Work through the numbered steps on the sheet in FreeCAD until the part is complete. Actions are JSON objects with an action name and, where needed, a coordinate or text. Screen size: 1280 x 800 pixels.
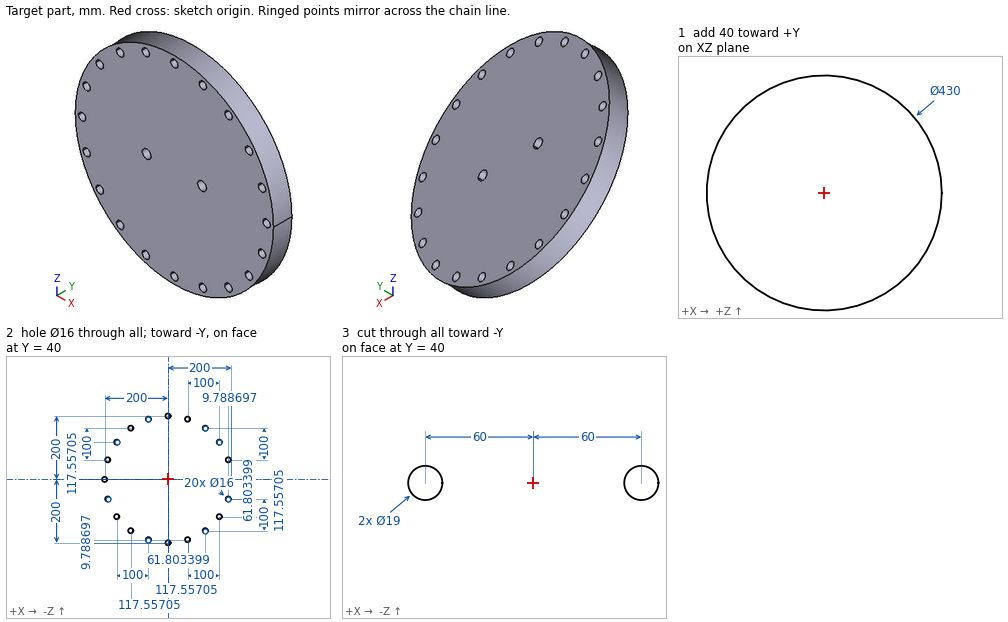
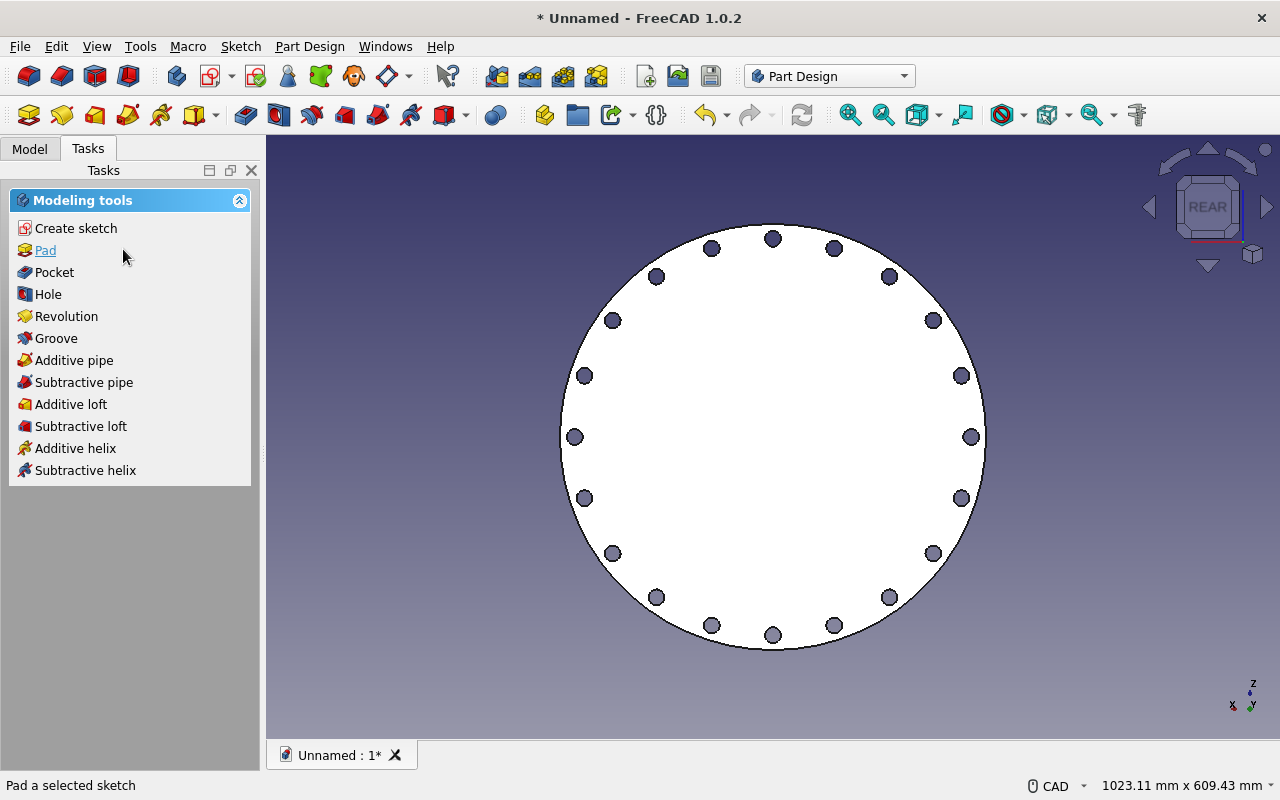
{"action": "left_click", "coordinate": [246, 116]}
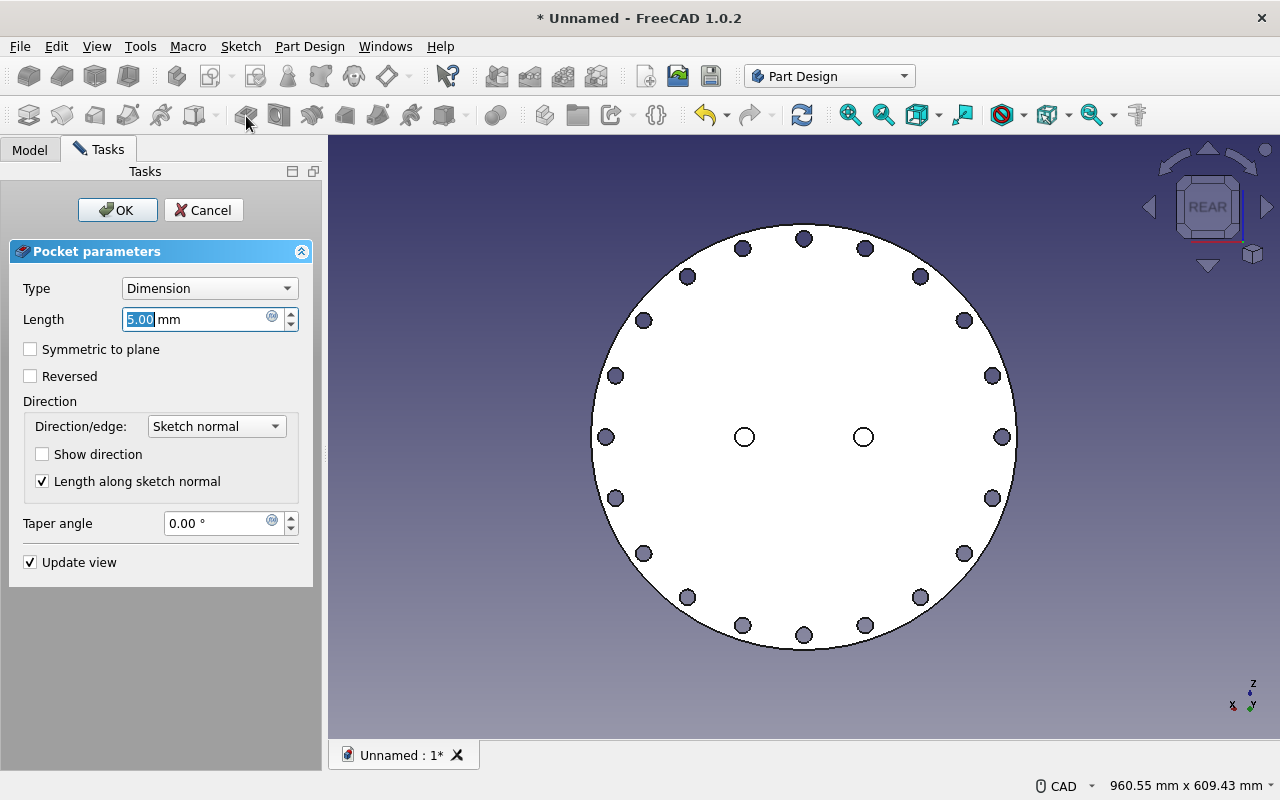
{"action": "left_click", "coordinate": [210, 288]}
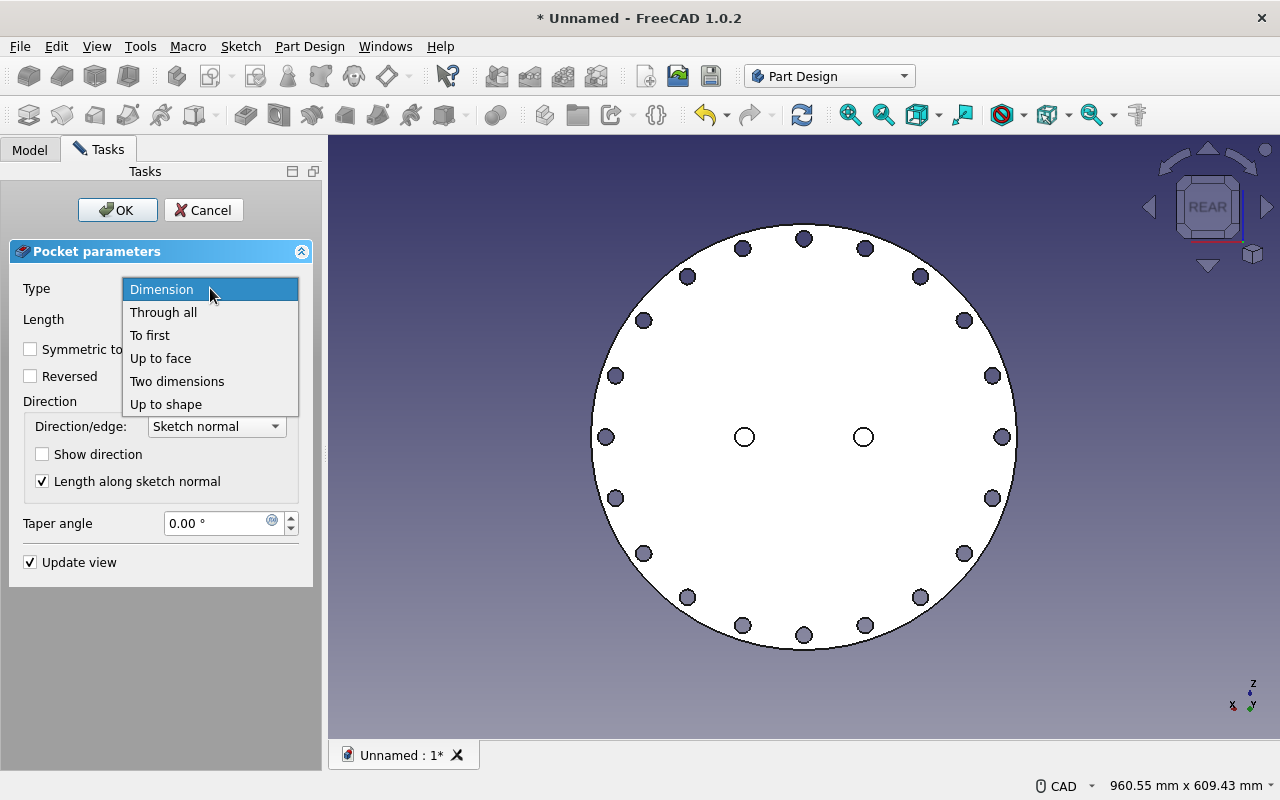
{"action": "left_click", "coordinate": [208, 312]}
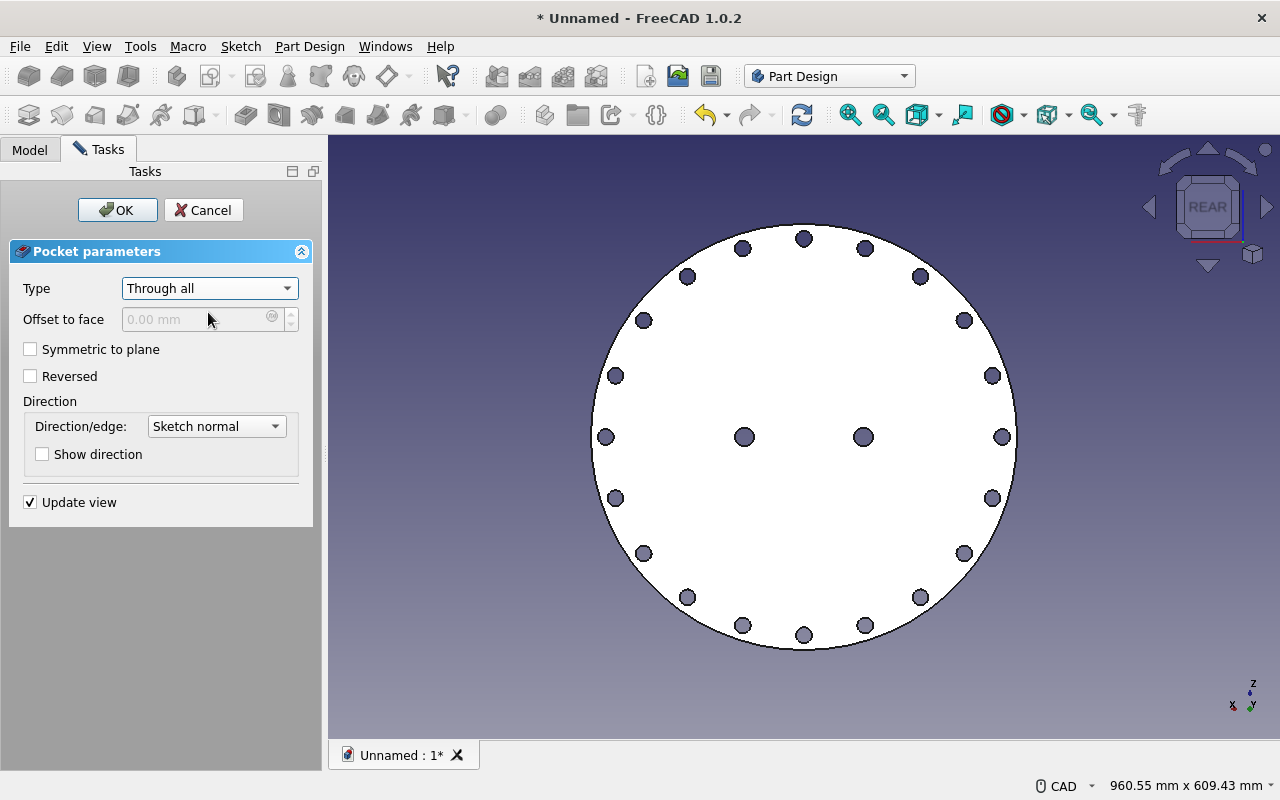
{"action": "left_click", "coordinate": [118, 210]}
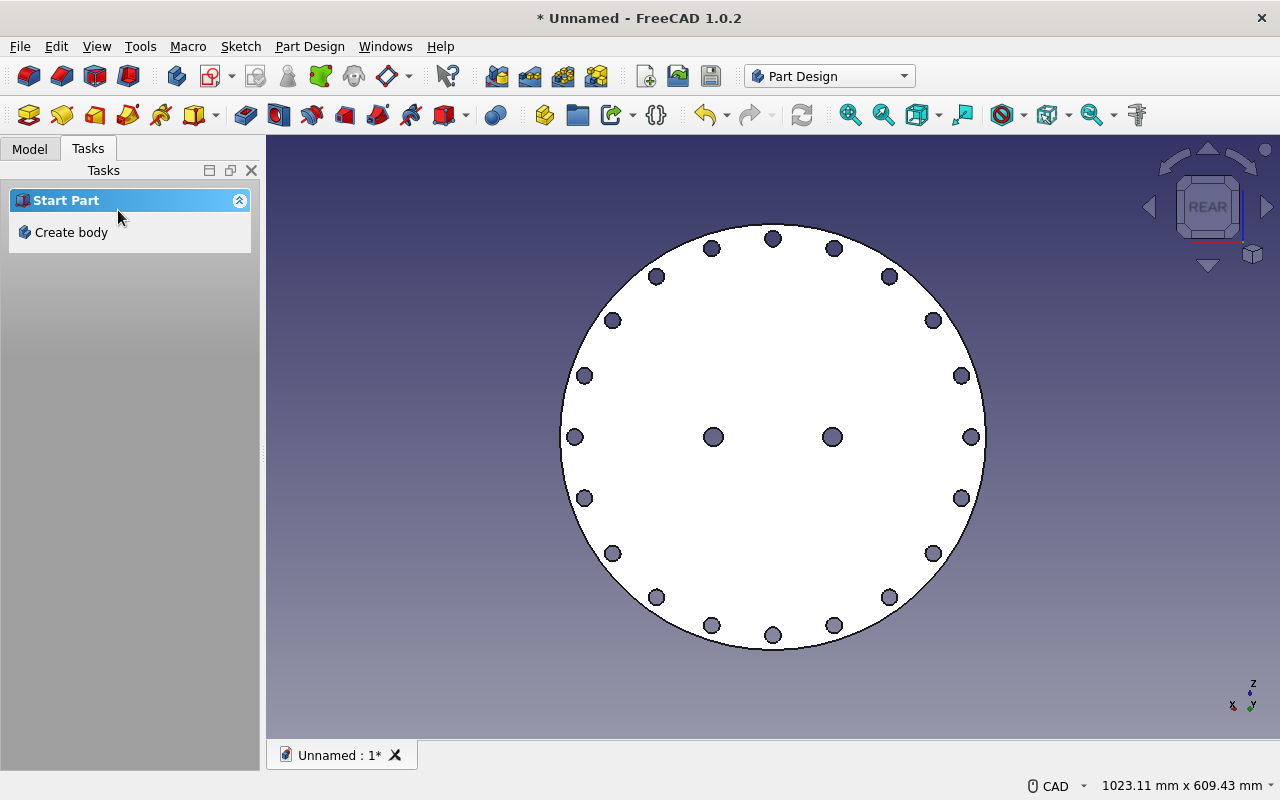
{"action": "key", "text": "0"}